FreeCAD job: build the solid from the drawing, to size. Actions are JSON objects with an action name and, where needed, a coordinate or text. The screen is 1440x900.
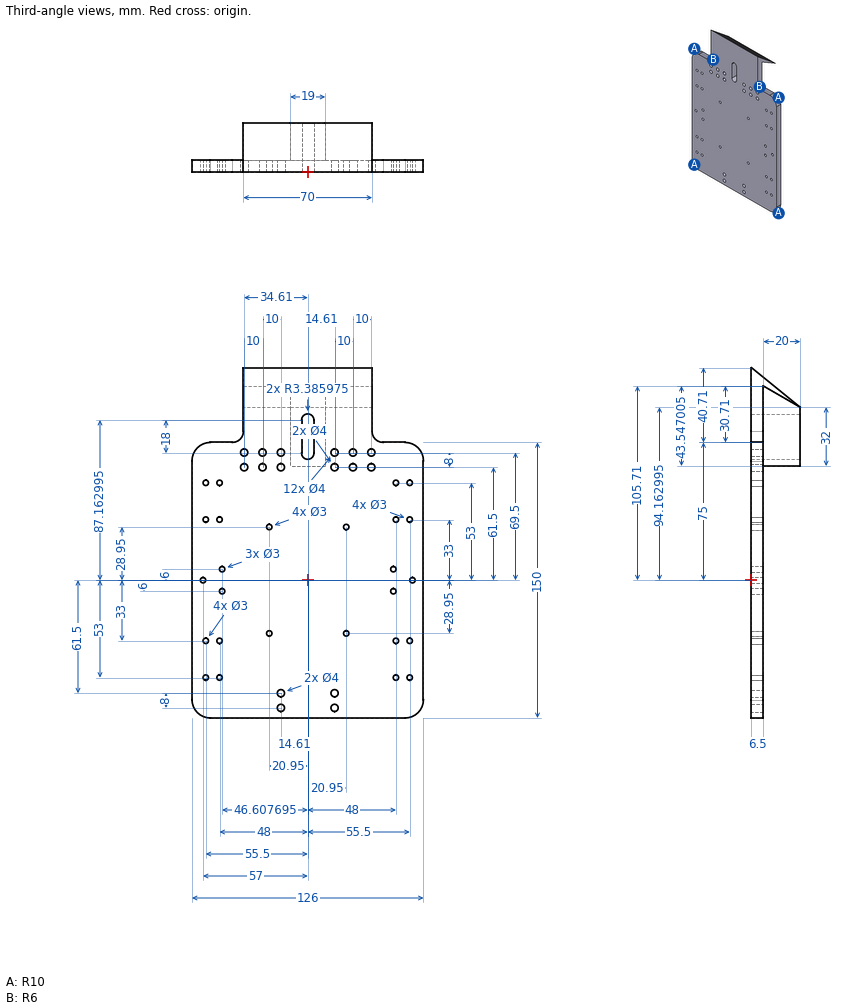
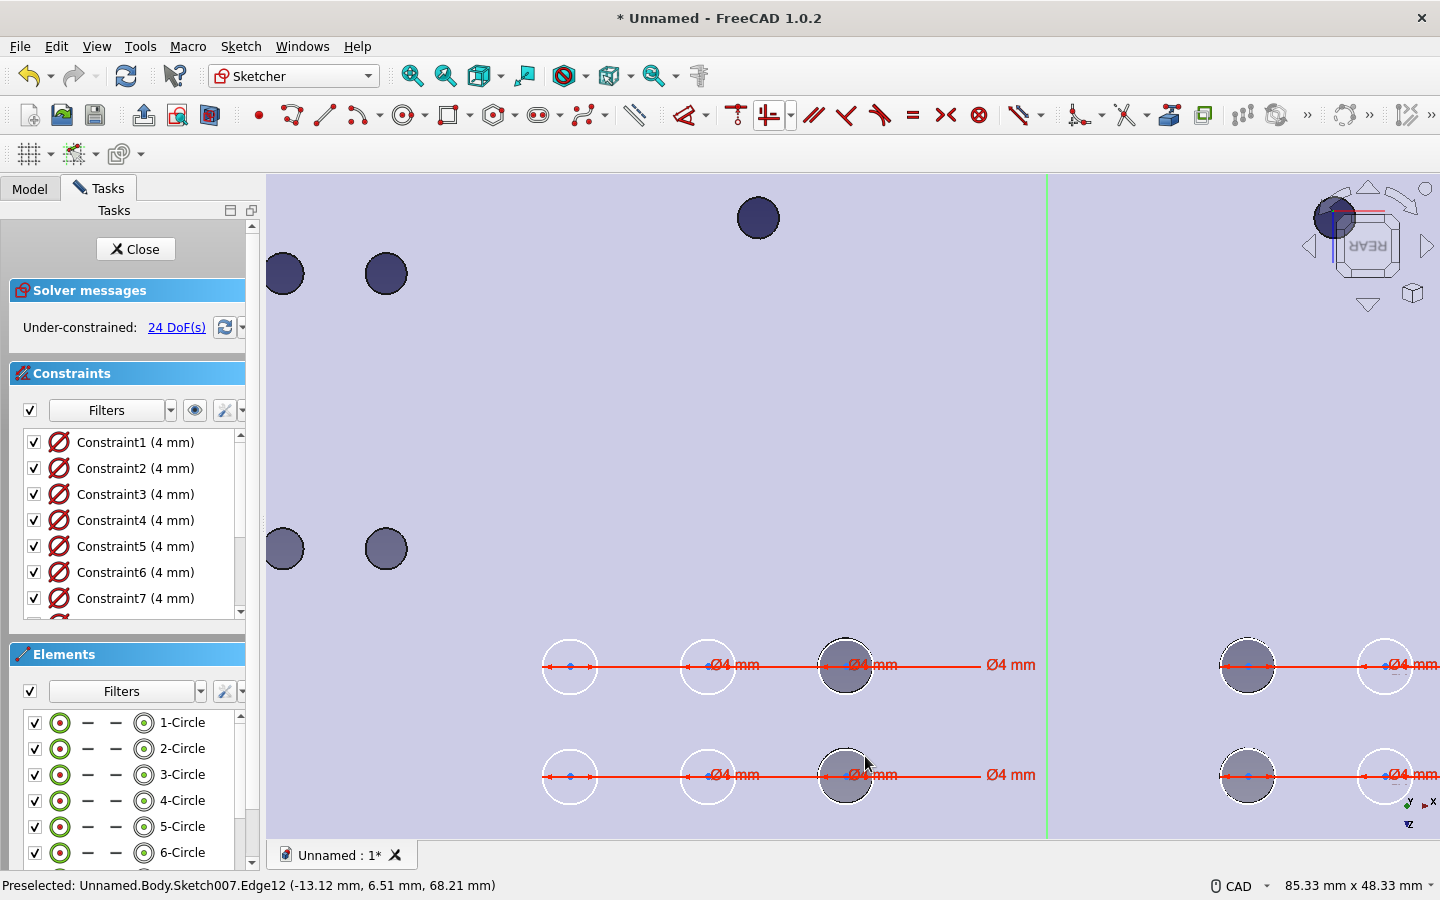
{"action": "left_click", "coordinate": [1248, 777]}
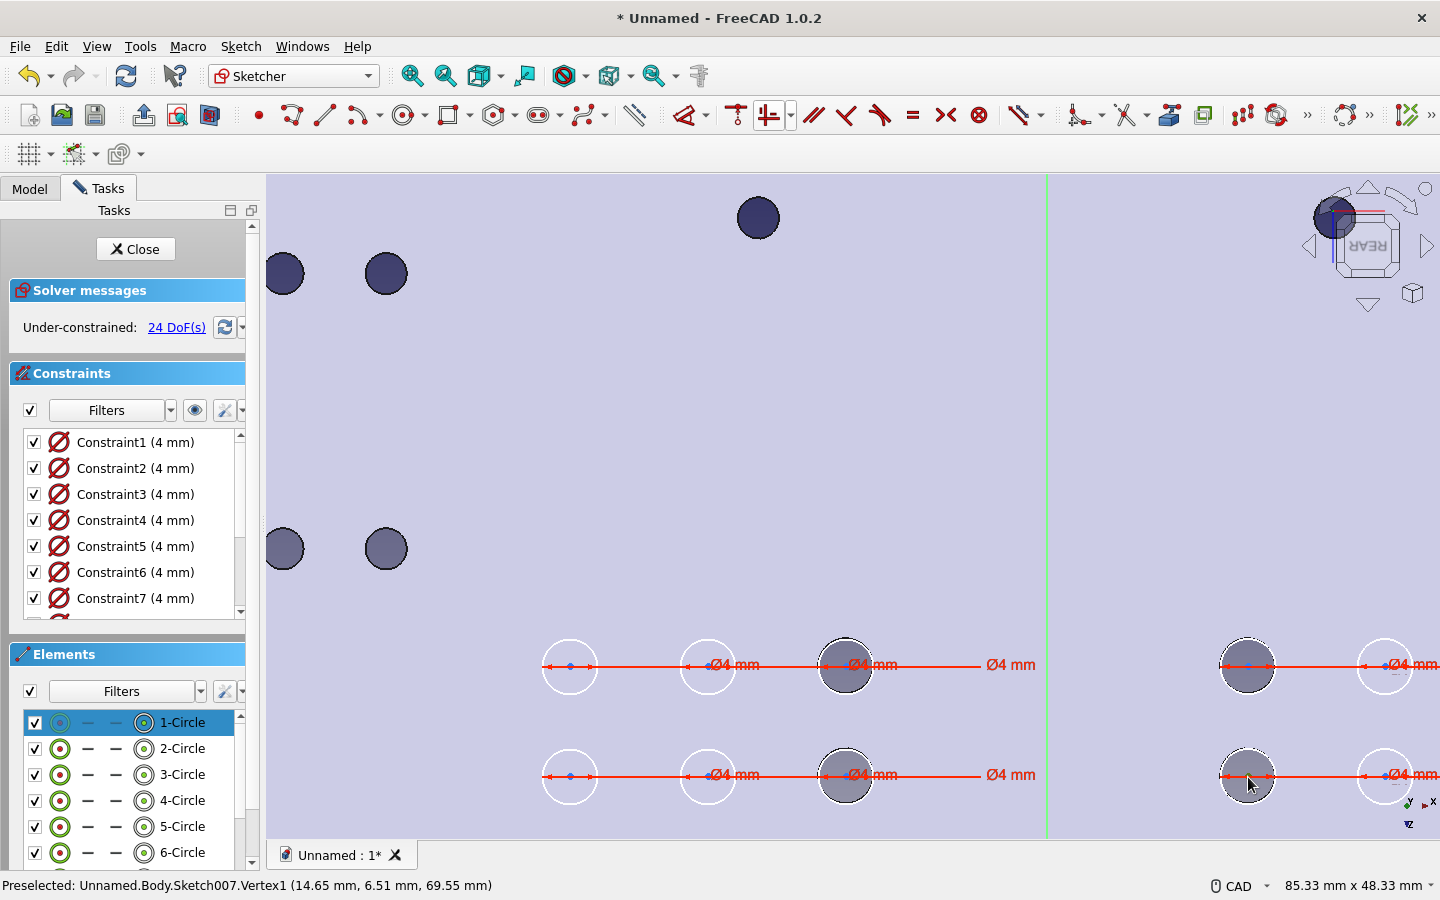
{"action": "left_click", "coordinate": [1248, 667]}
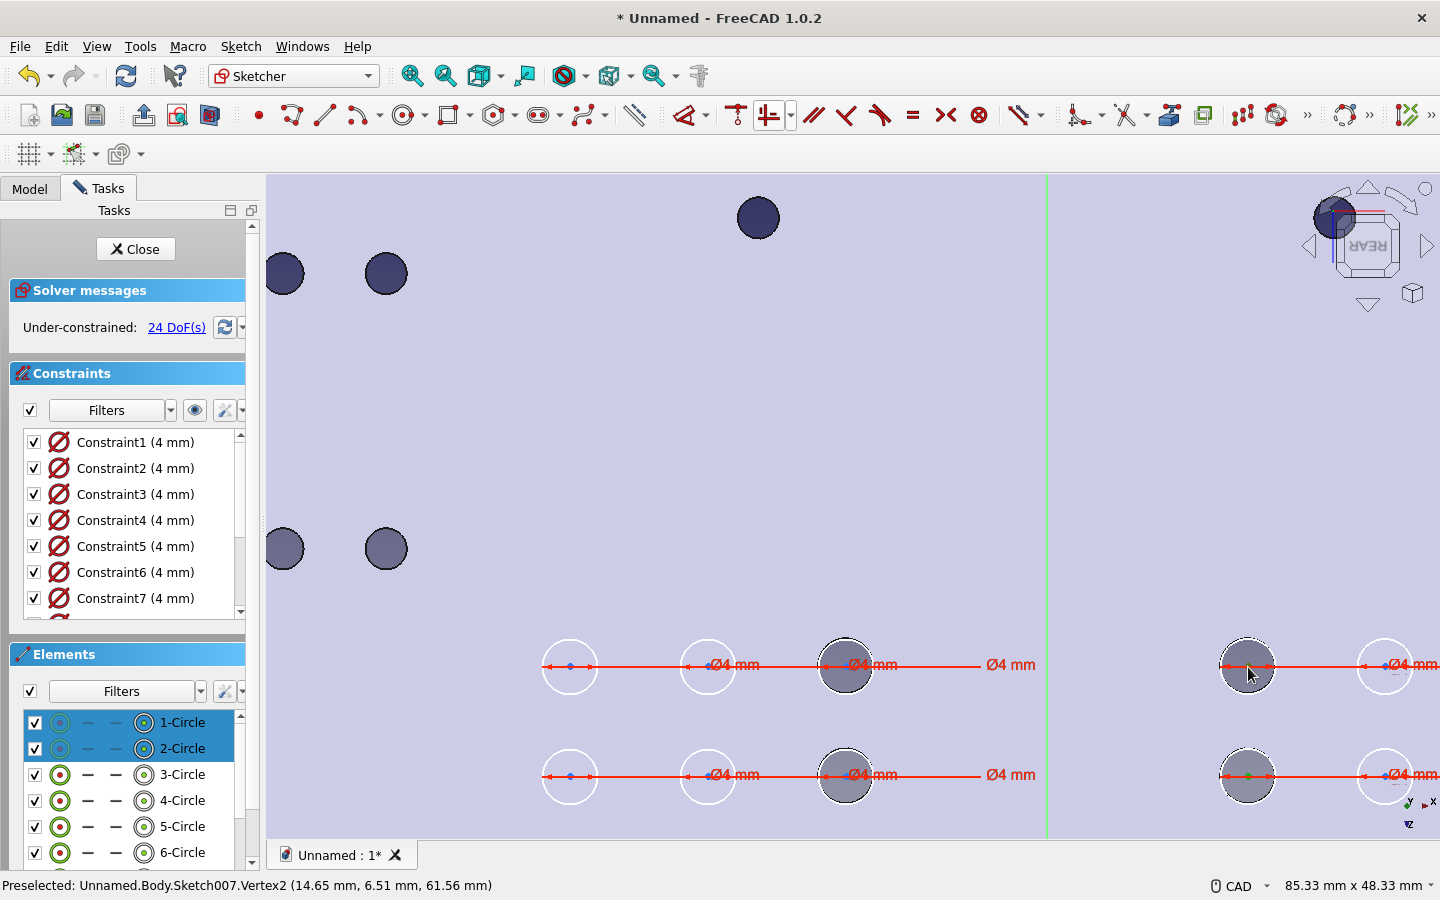
{"action": "left_click", "coordinate": [790, 116]}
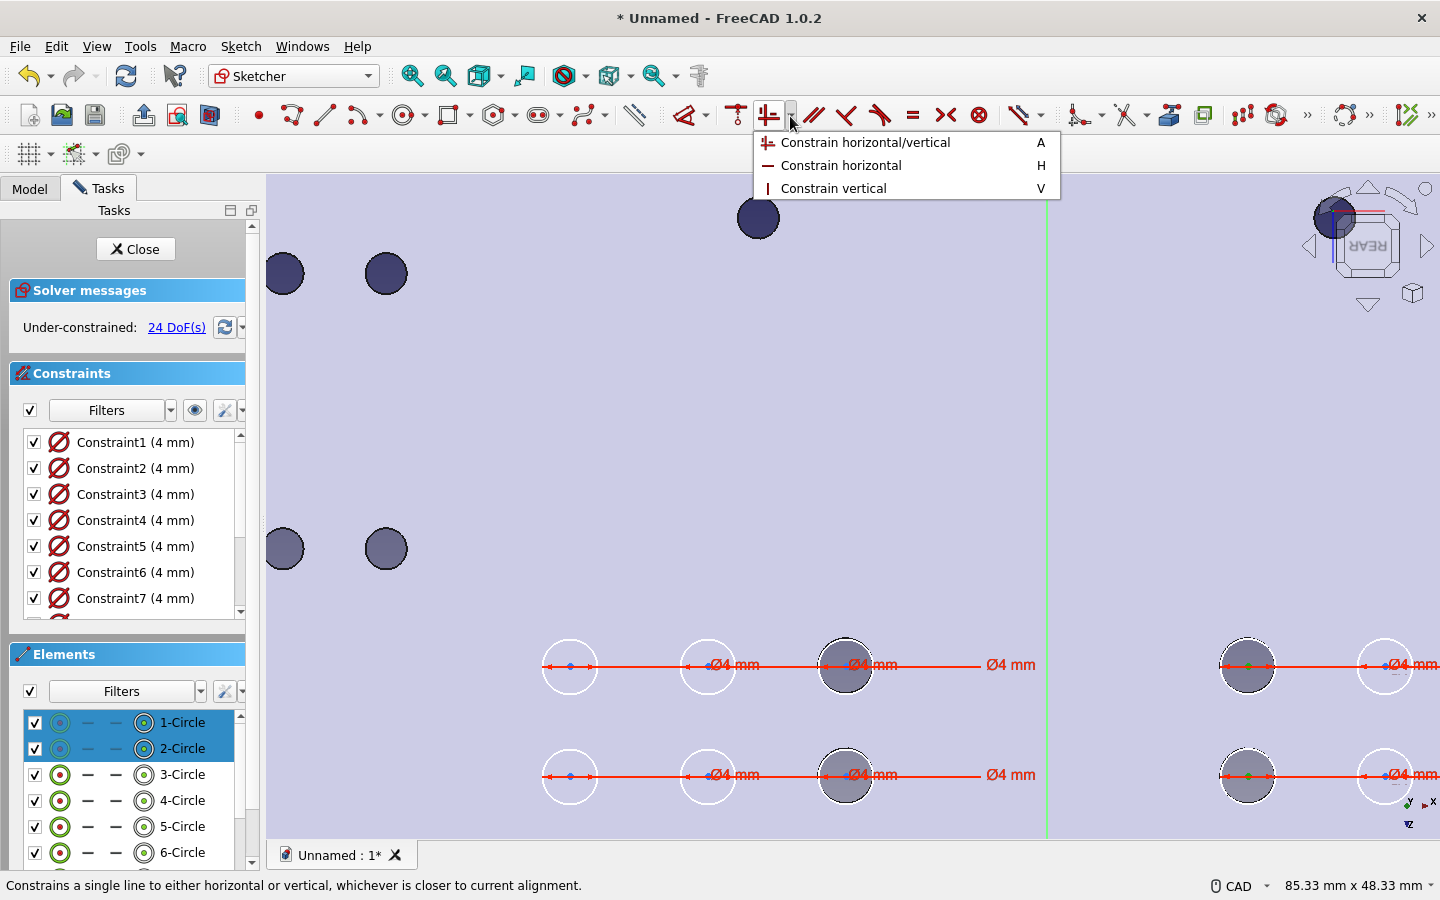
{"action": "left_click", "coordinate": [907, 188]}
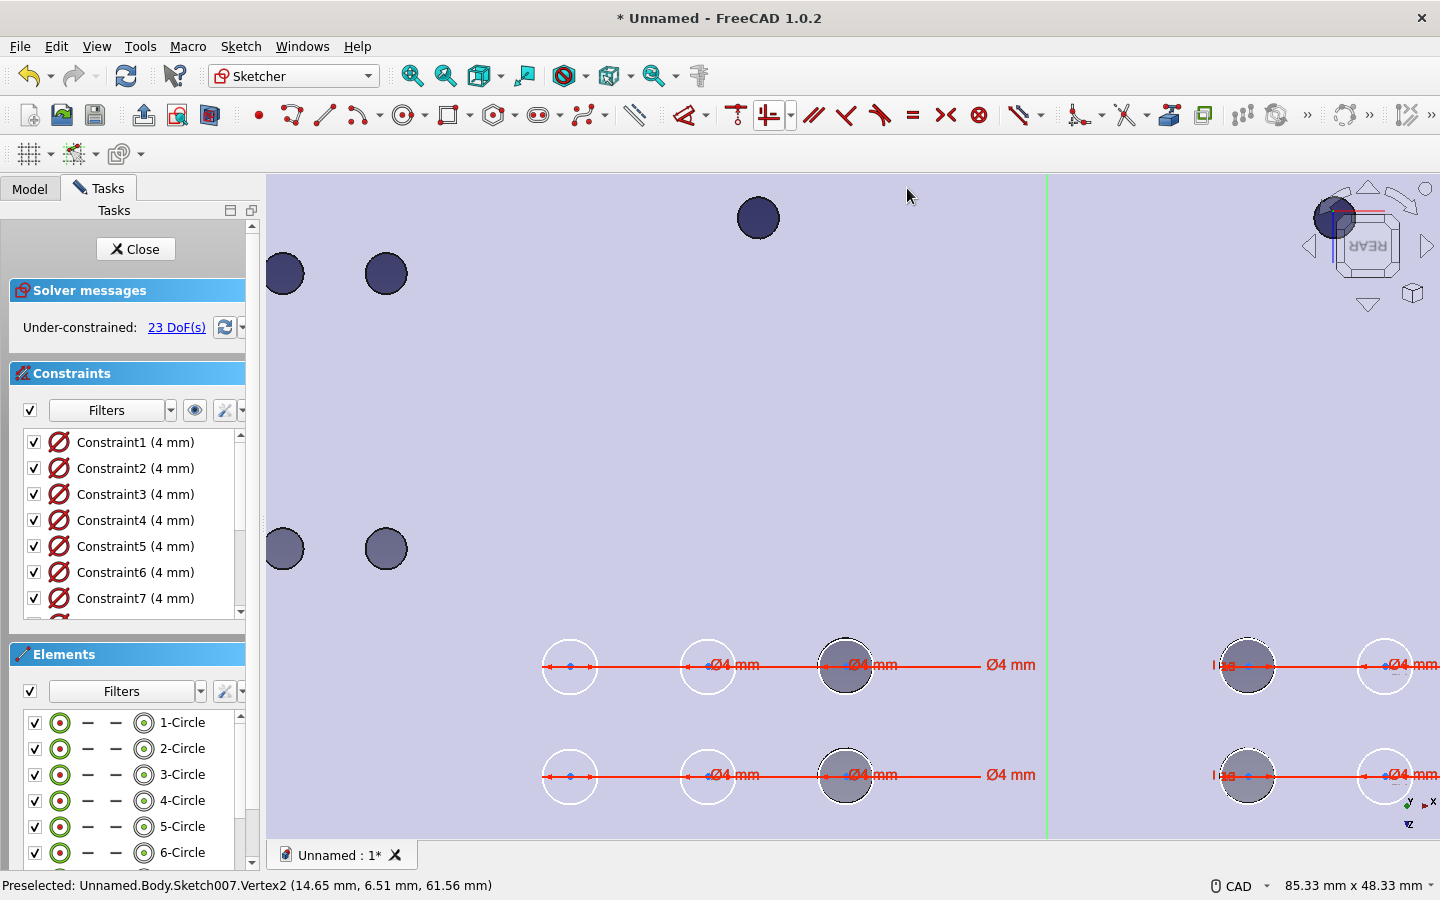
{"action": "left_click", "coordinate": [1248, 777]}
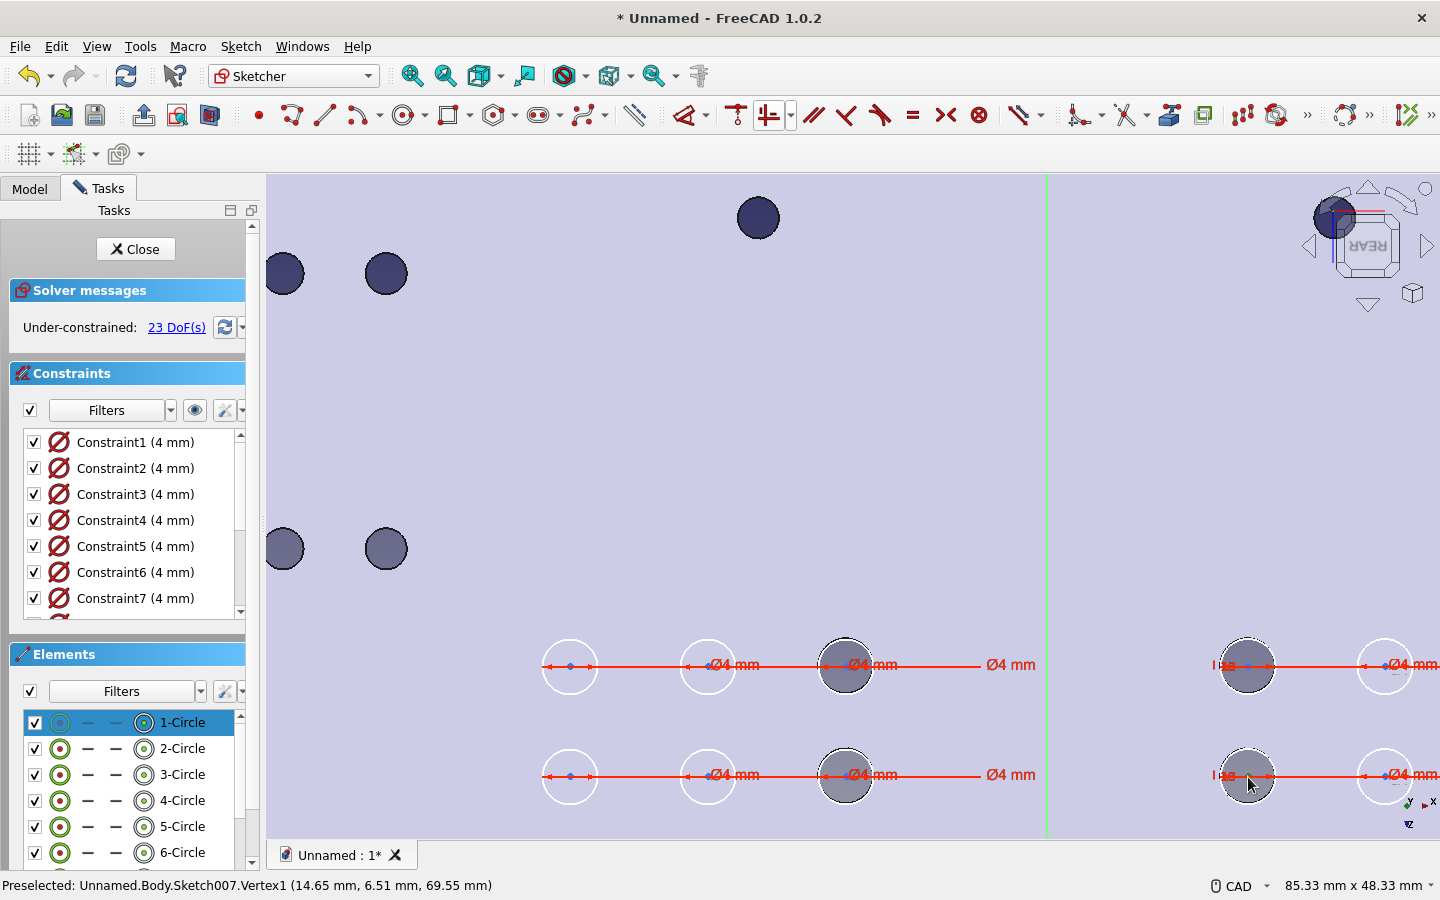
{"action": "scroll", "coordinate": [571, 666], "scroll_direction": "down", "scroll_amount": 4}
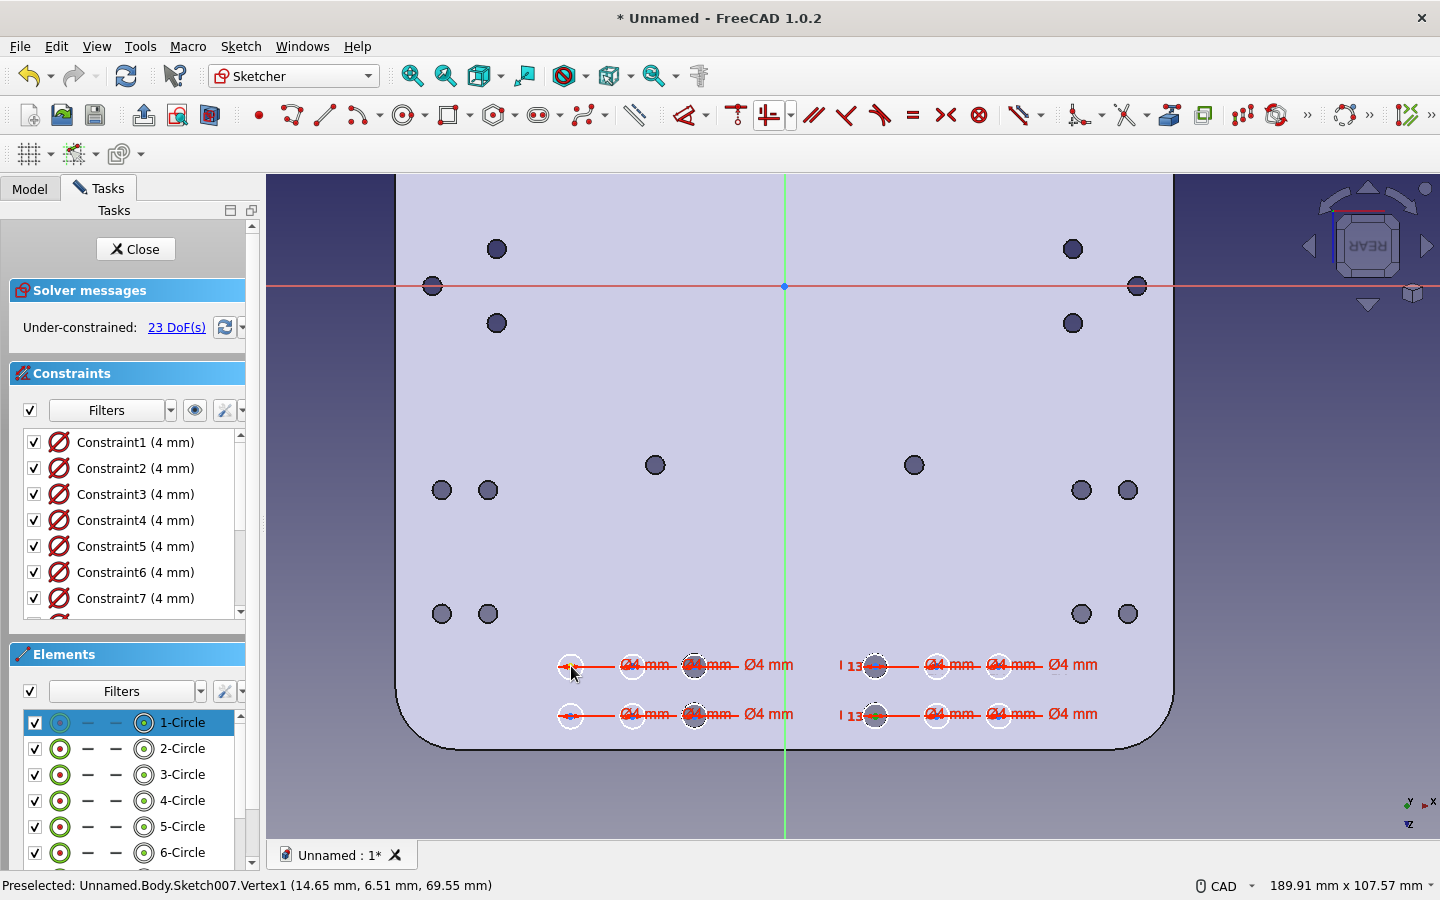
{"action": "left_click", "coordinate": [937, 716]}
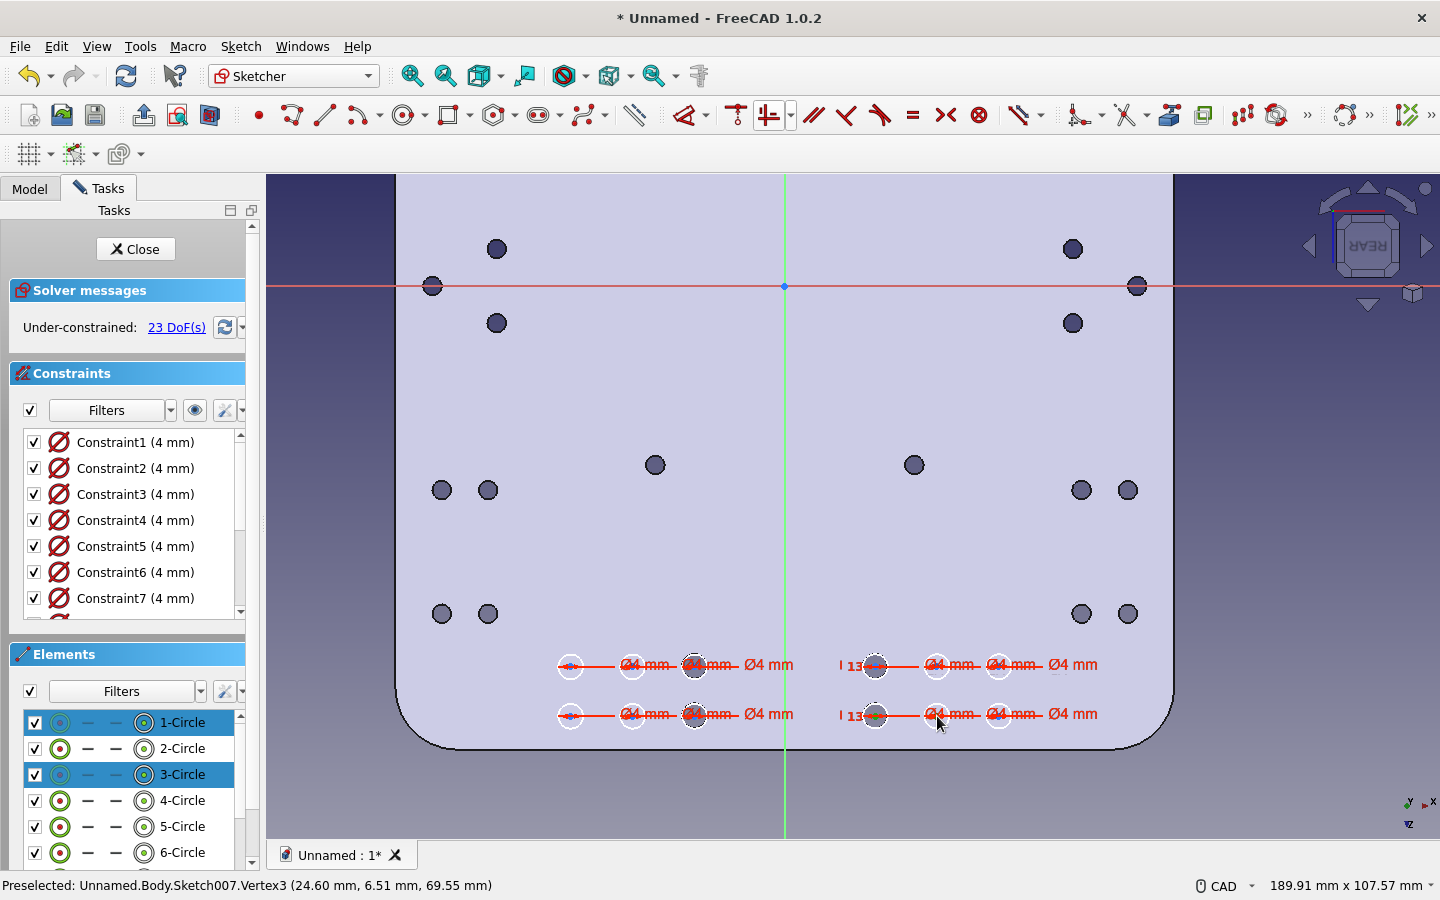
{"action": "key", "text": "h"}